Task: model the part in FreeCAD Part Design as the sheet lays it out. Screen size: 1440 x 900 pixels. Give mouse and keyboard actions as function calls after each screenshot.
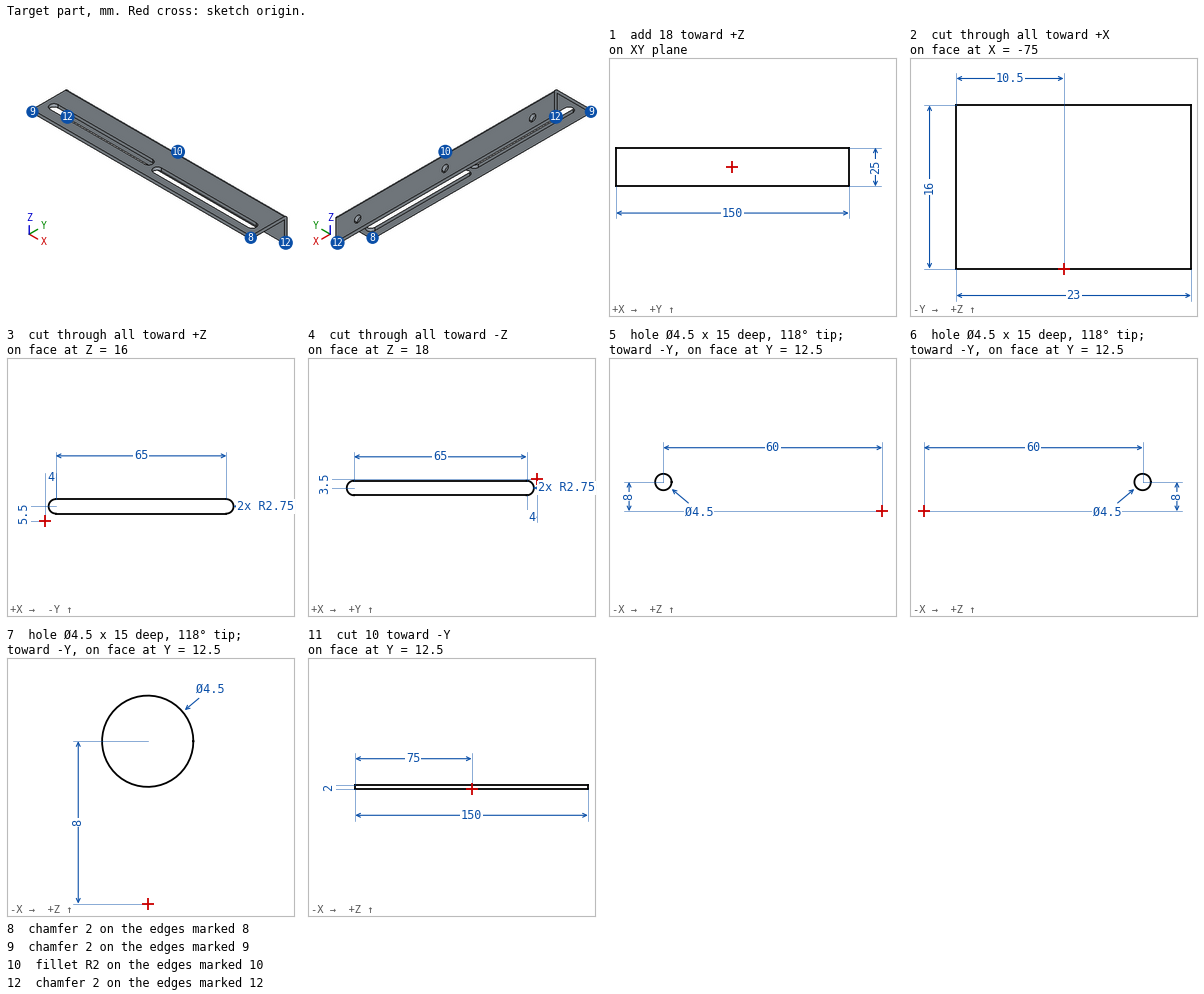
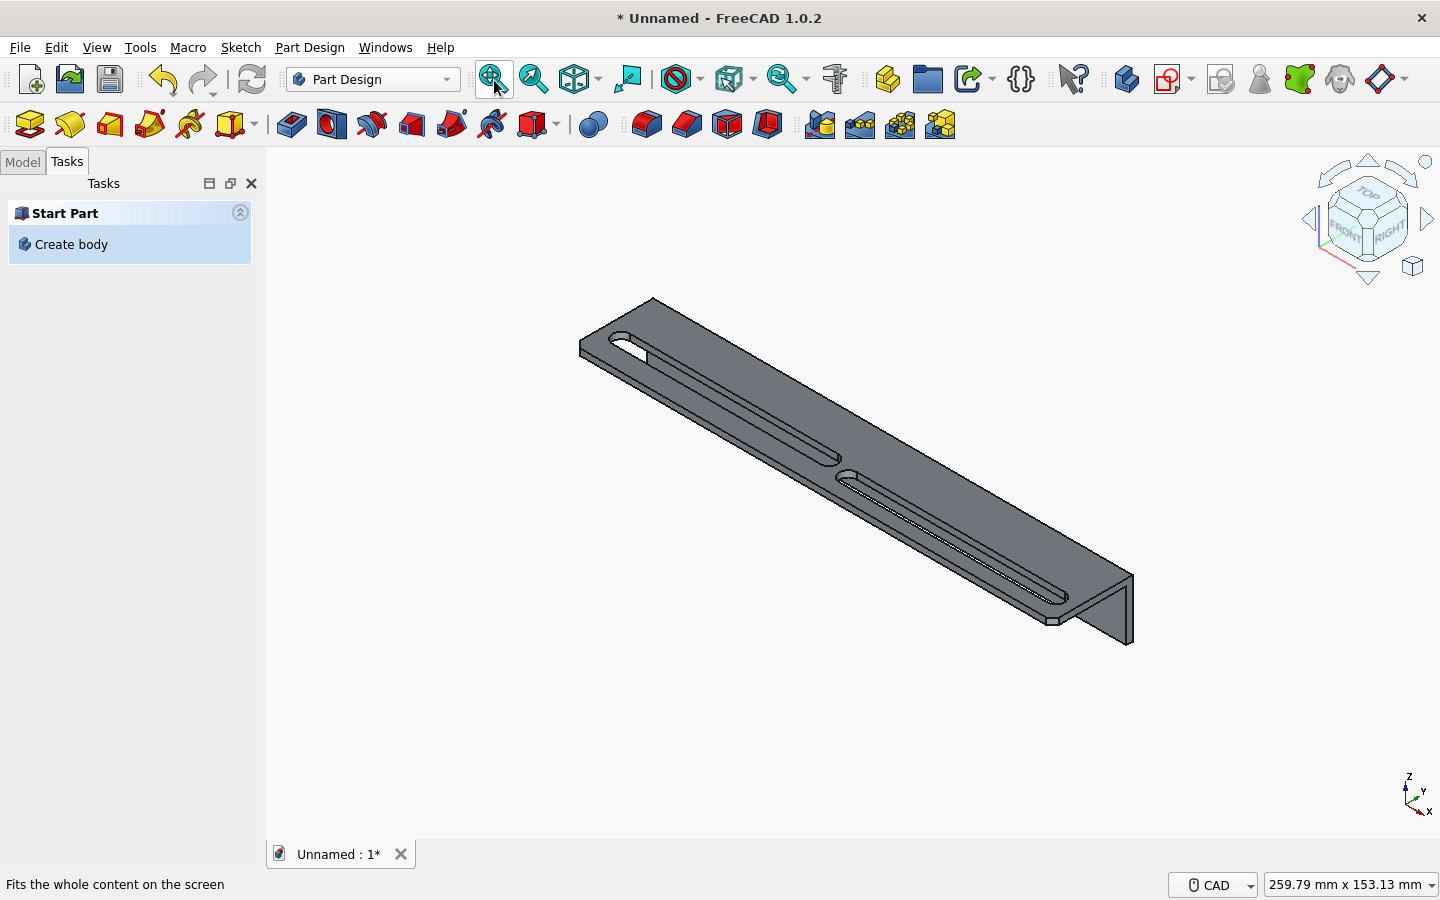
key(2)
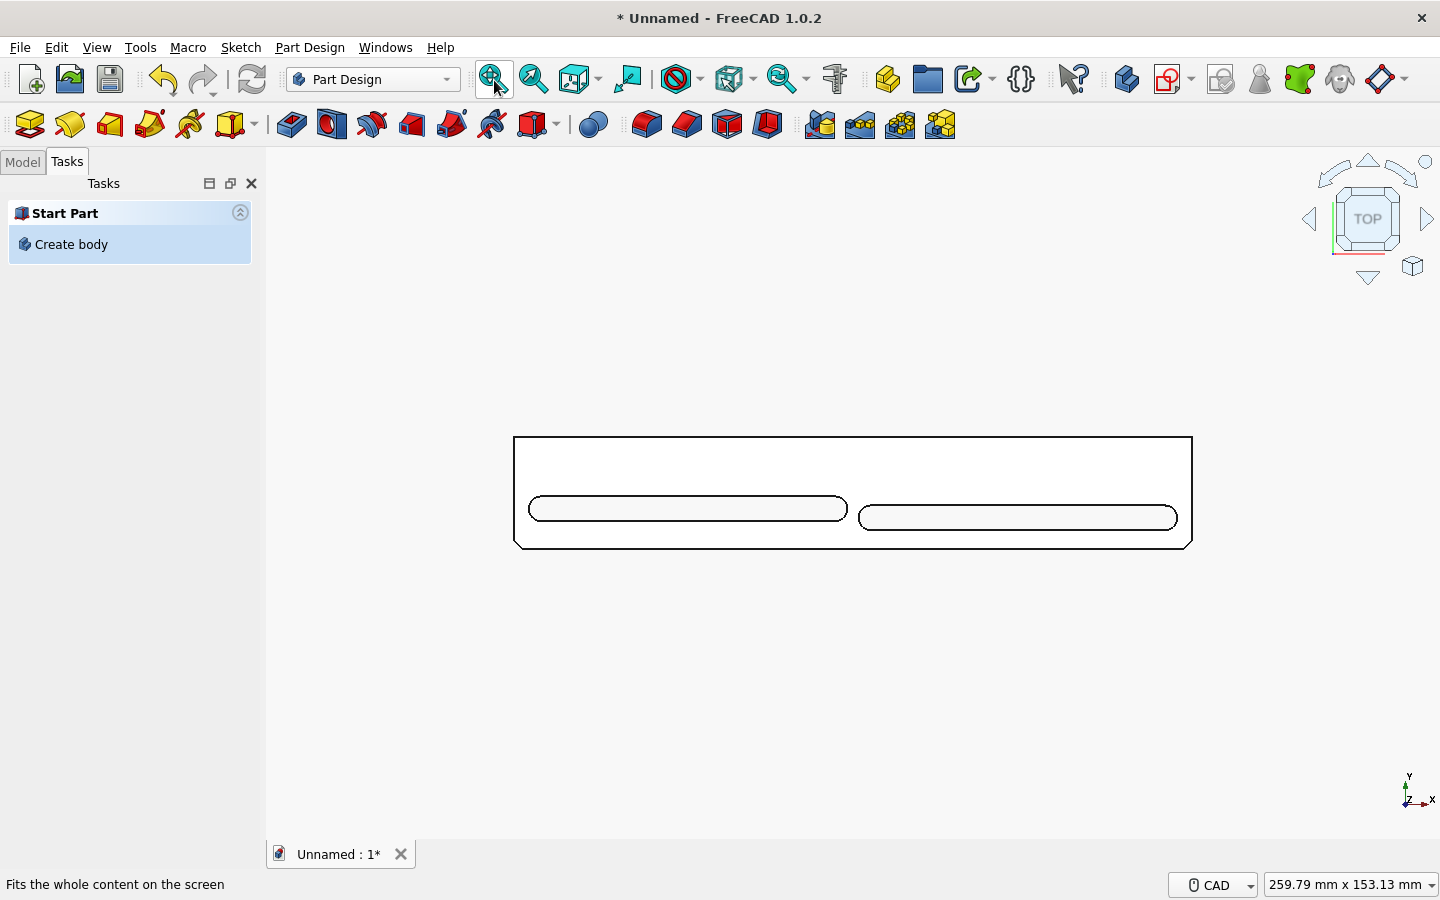
click(853, 436)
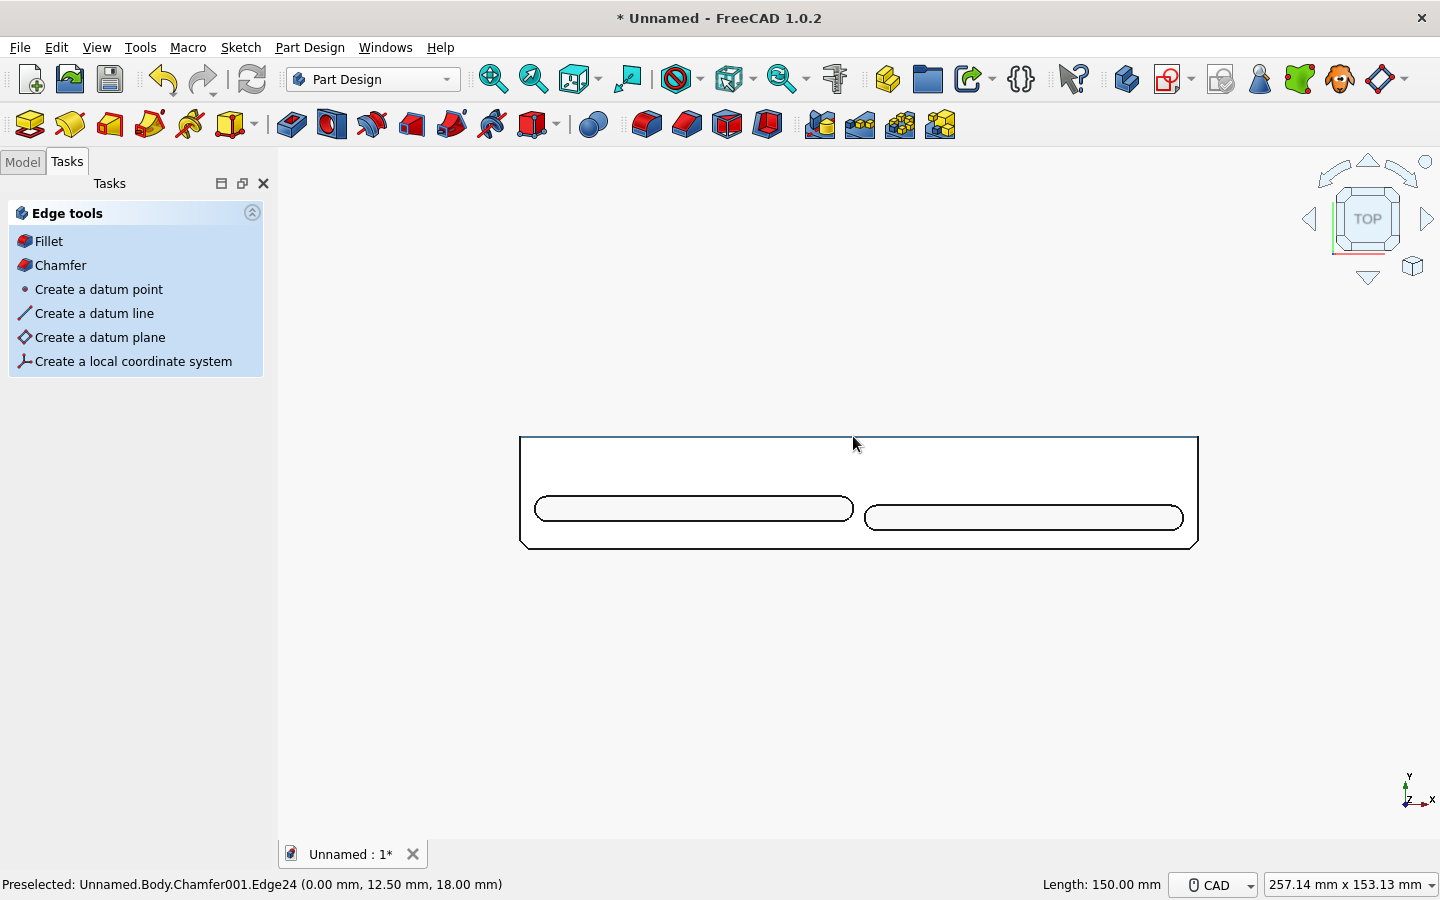
click(648, 124)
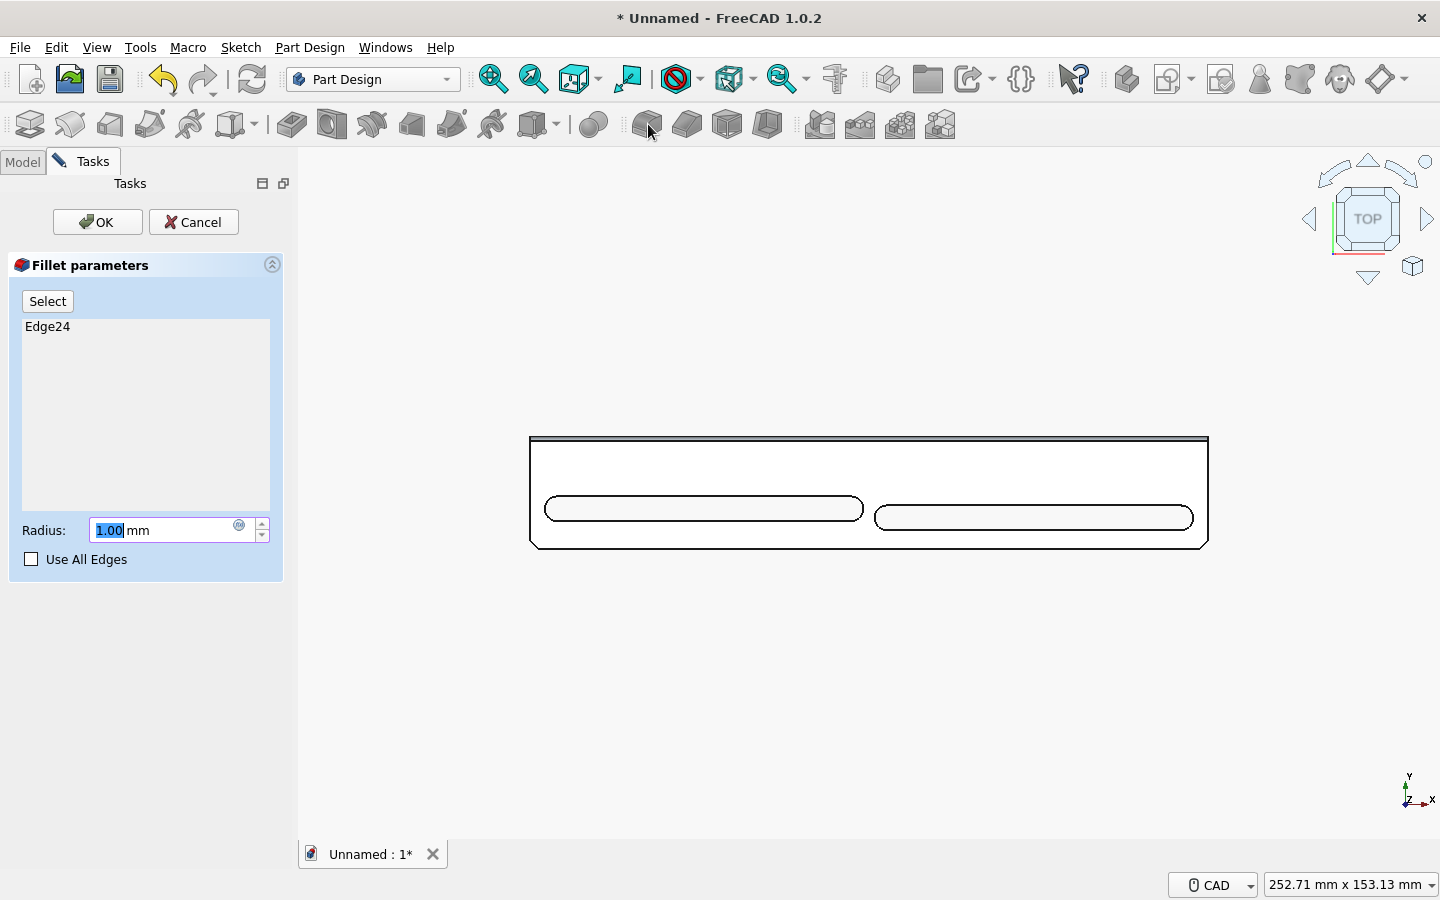
text(2)
key(Tab)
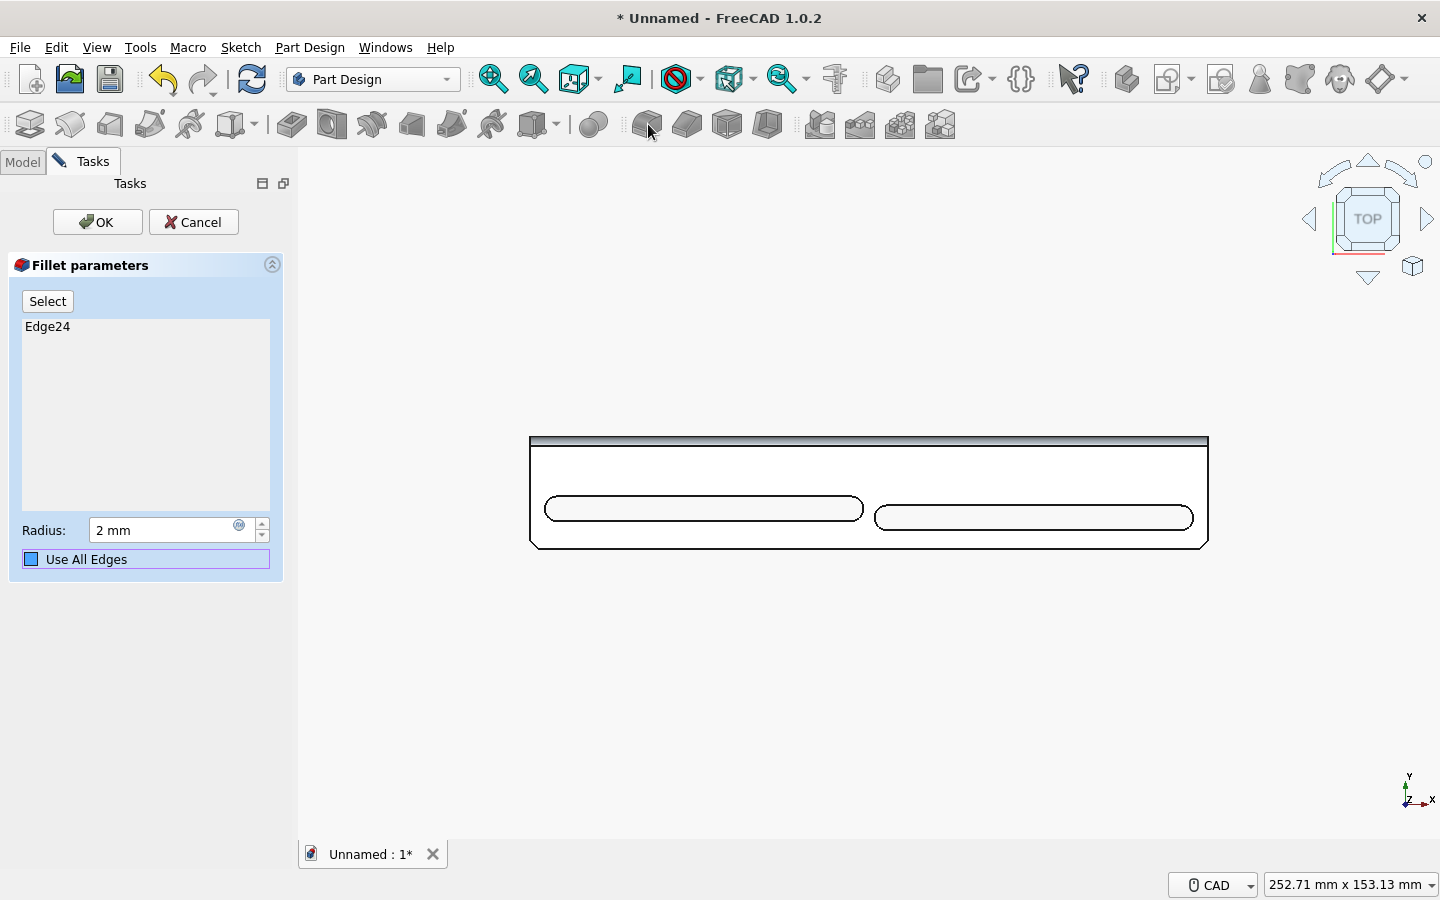
click(98, 222)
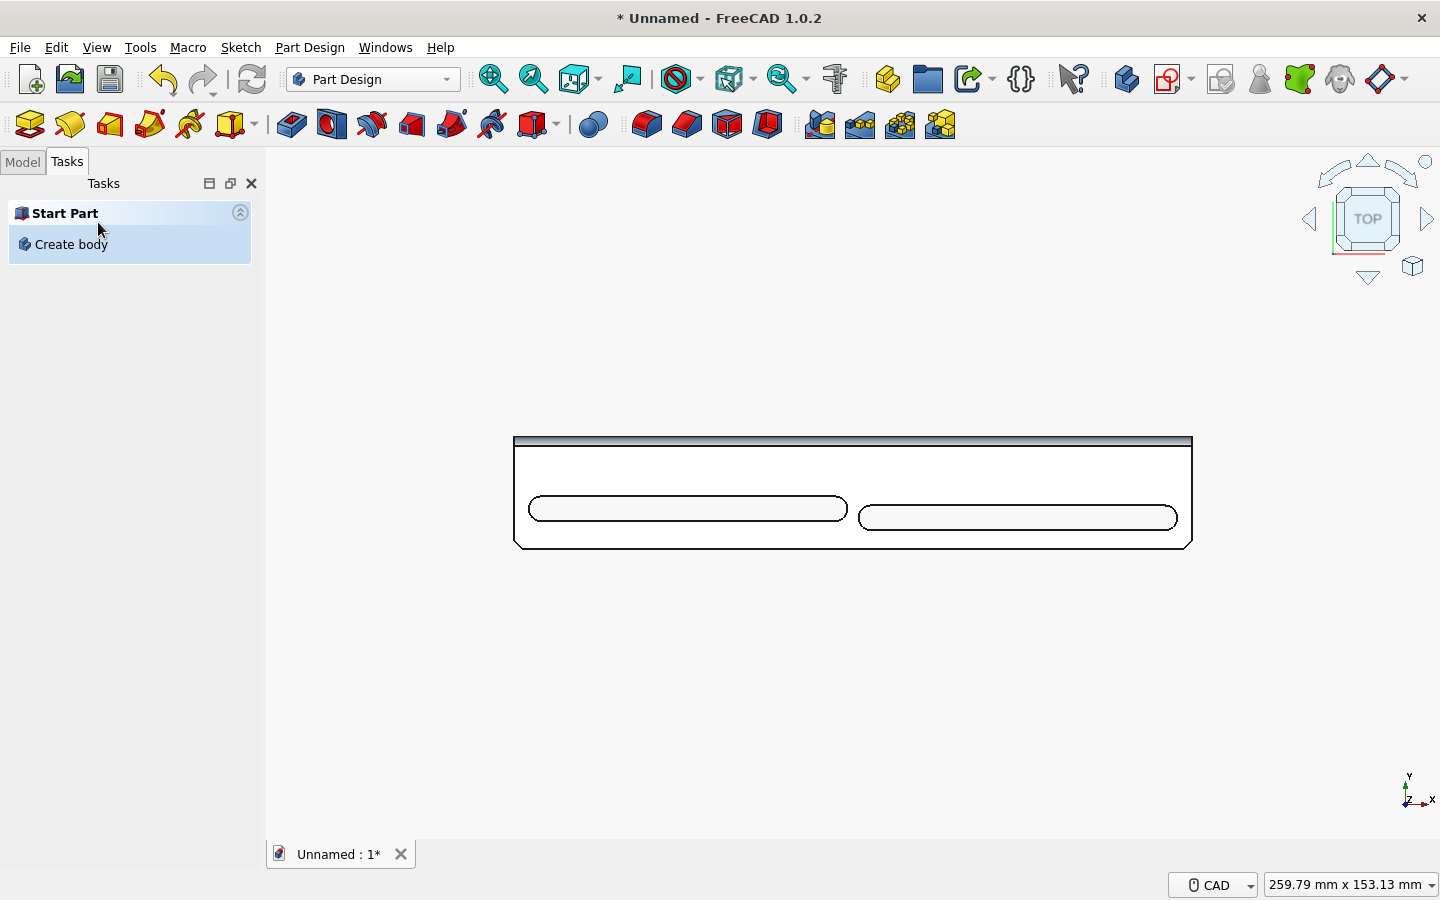
key(4)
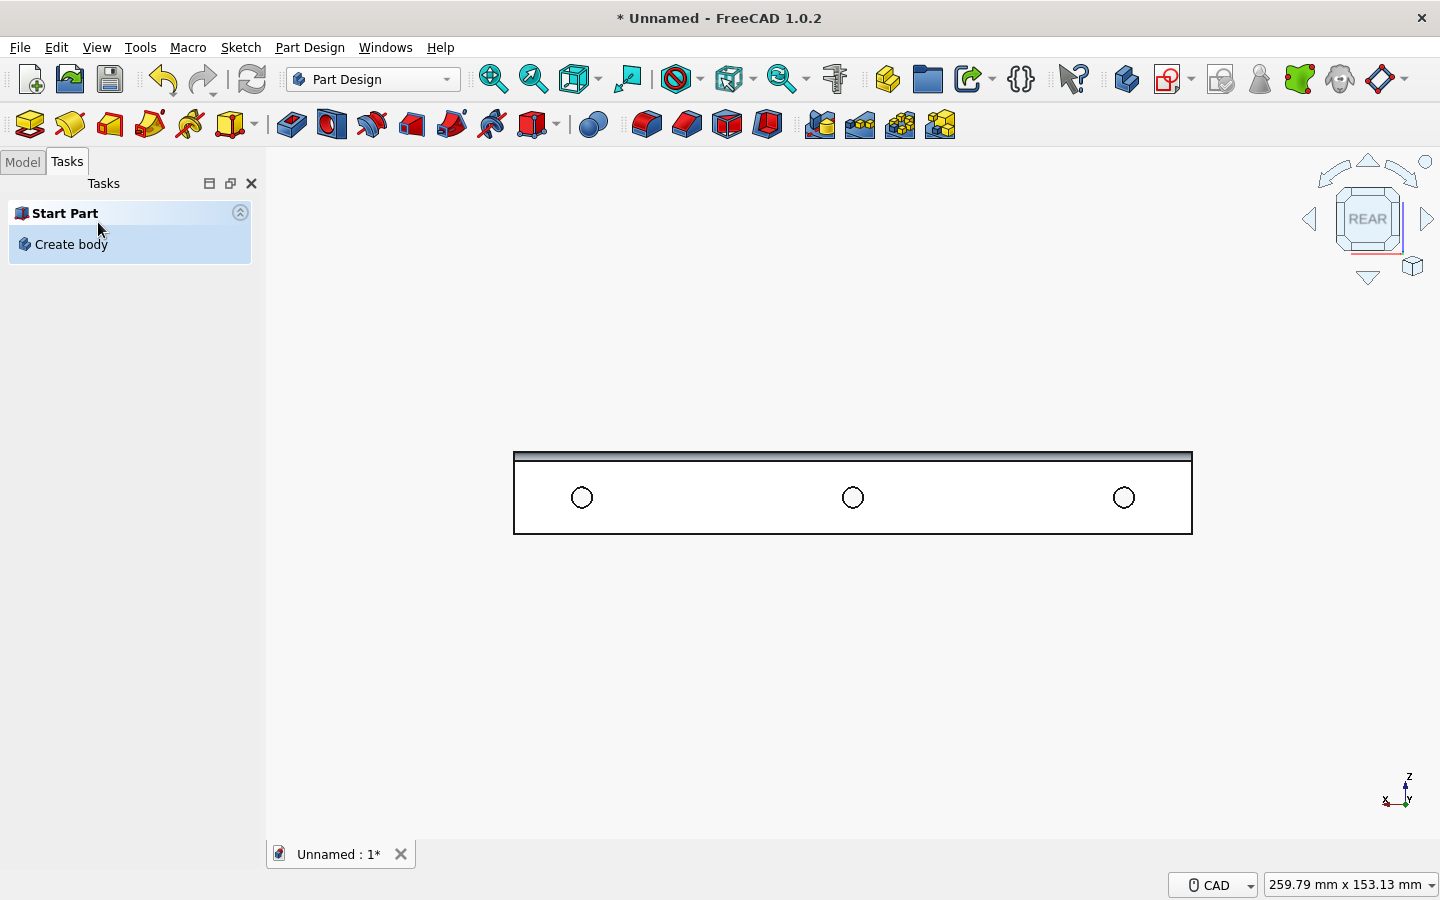
click(659, 497)